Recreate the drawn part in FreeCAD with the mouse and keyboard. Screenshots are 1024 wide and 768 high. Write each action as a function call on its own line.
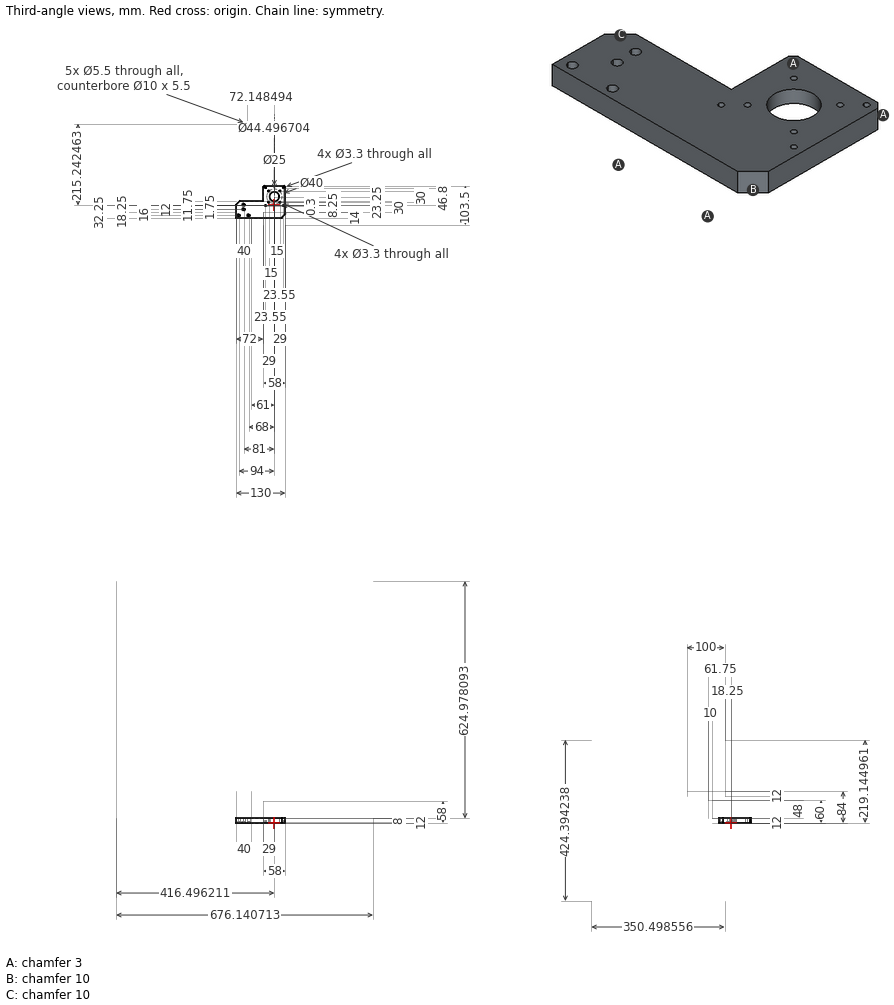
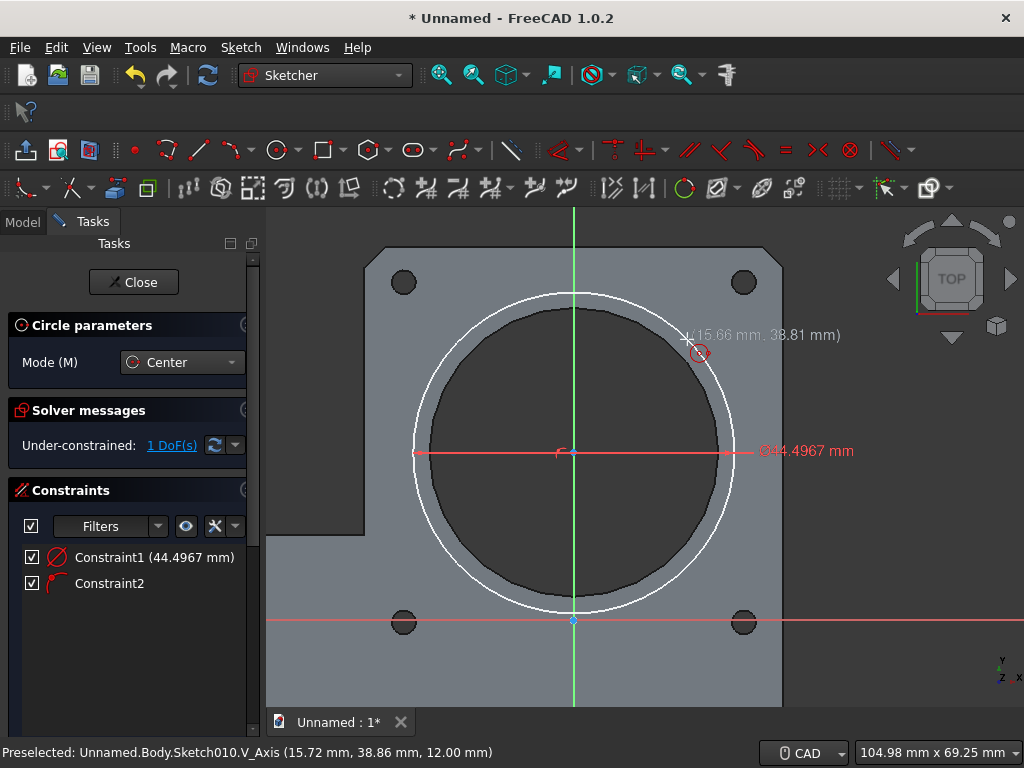
click(574, 453)
move(638, 389)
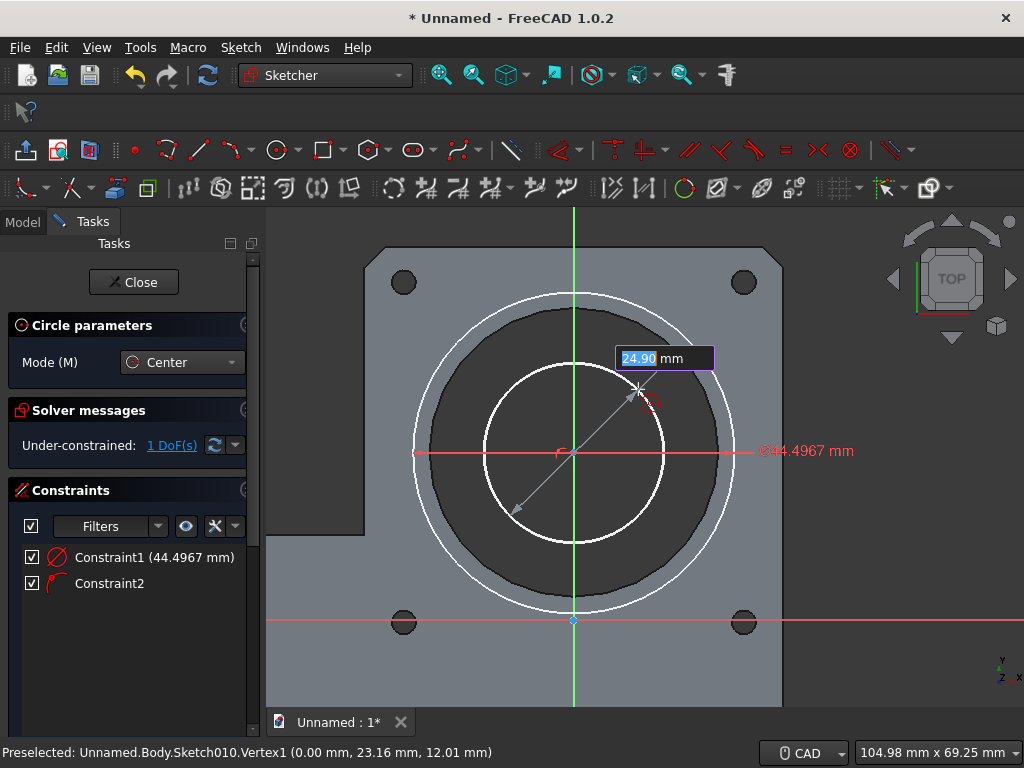
text(25)
key(Return)
key(Escape)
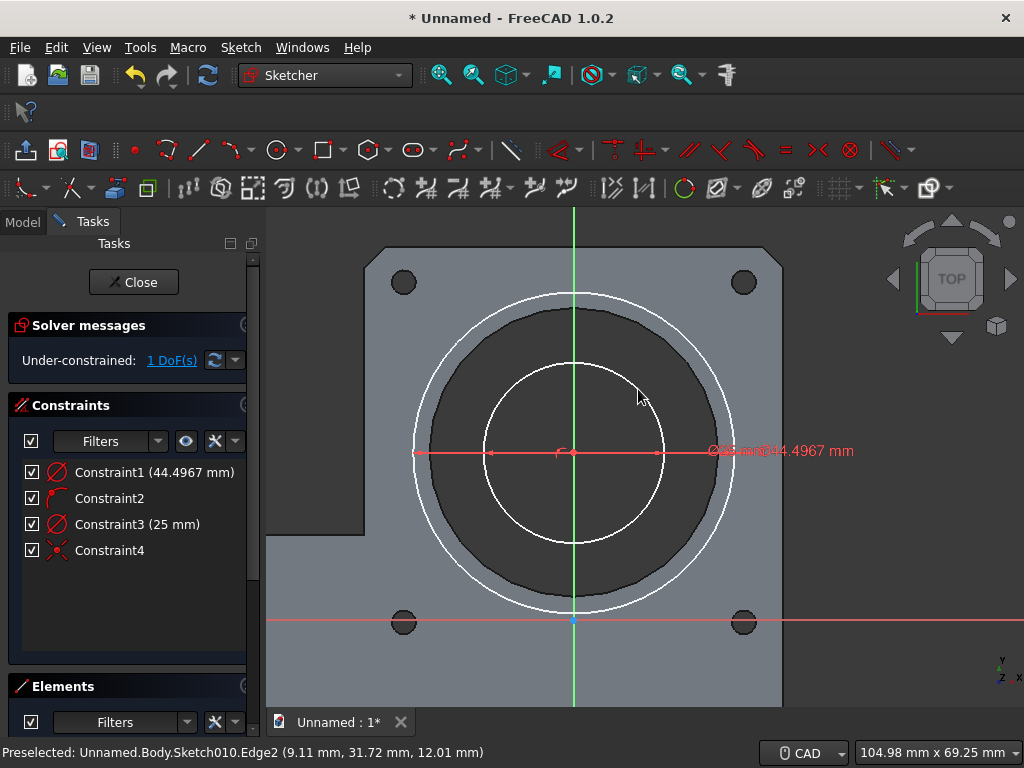
click(558, 150)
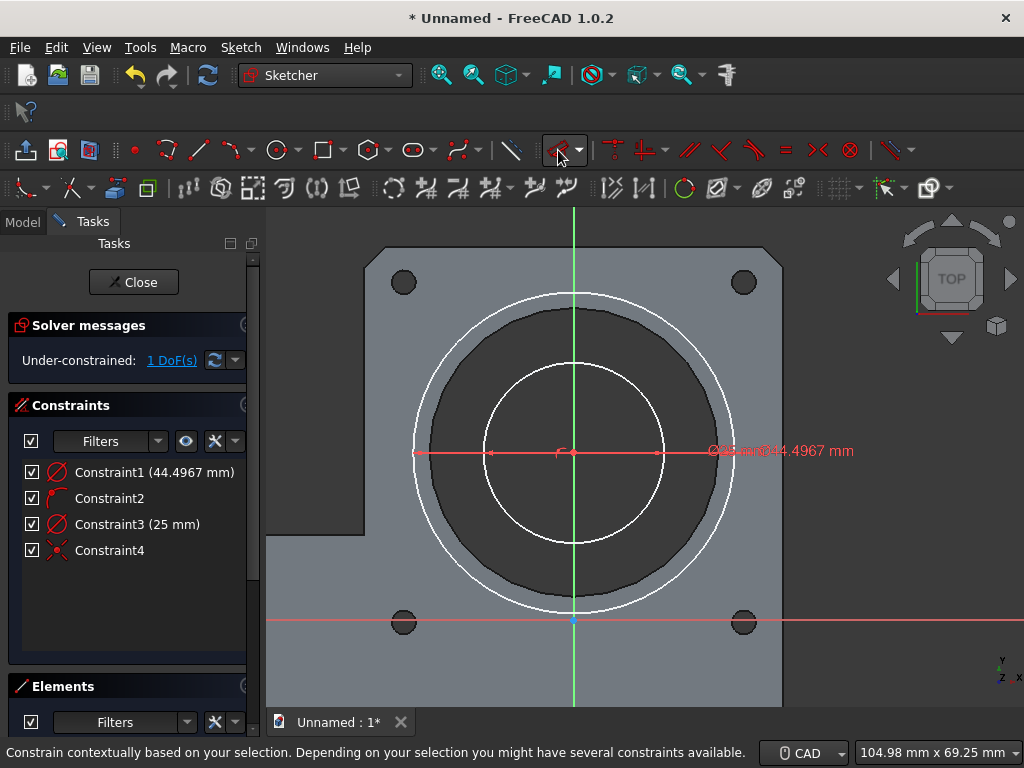
click(574, 453)
click(608, 498)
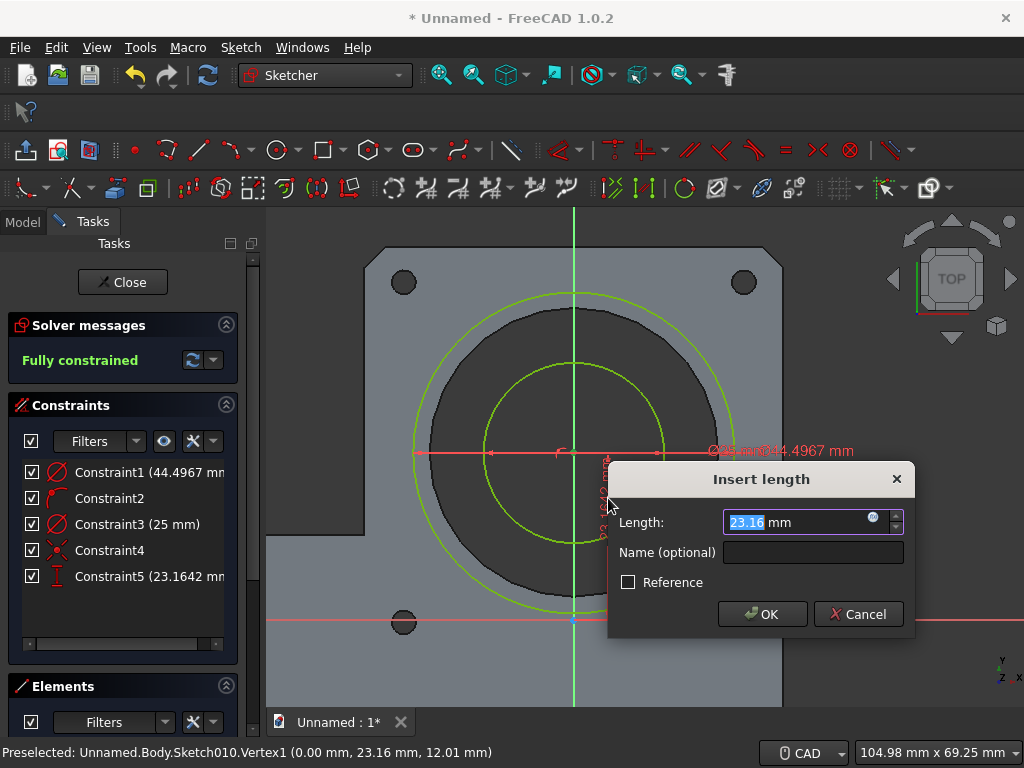
text(23.25)
key(Return)
key(Escape)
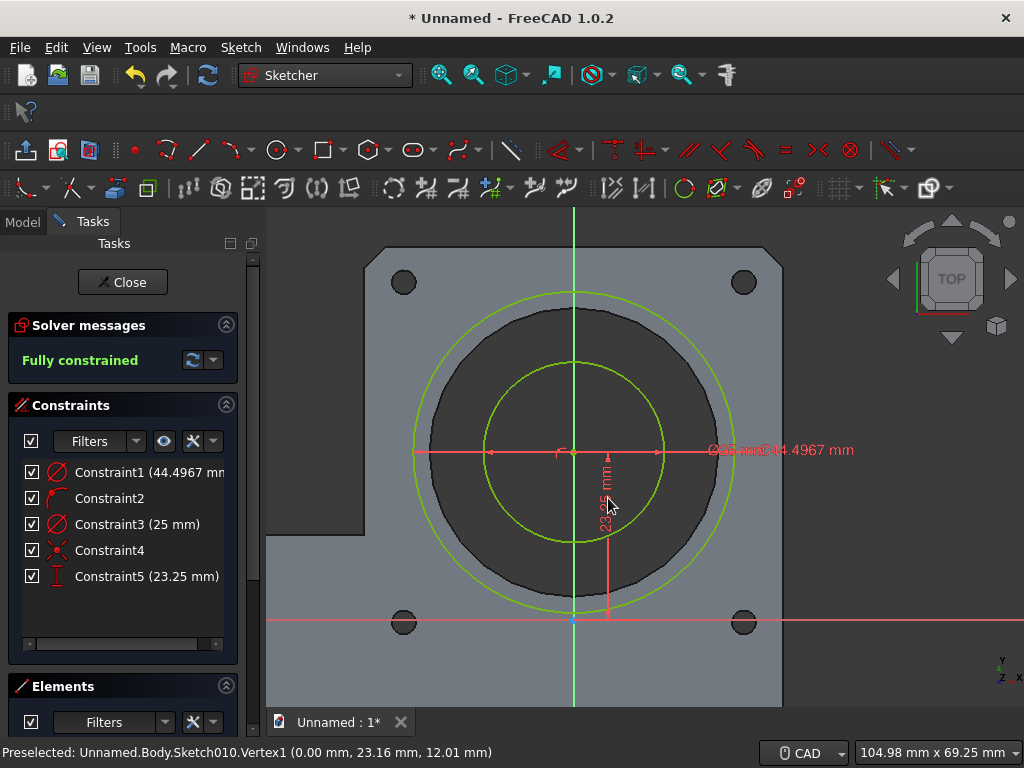
click(123, 282)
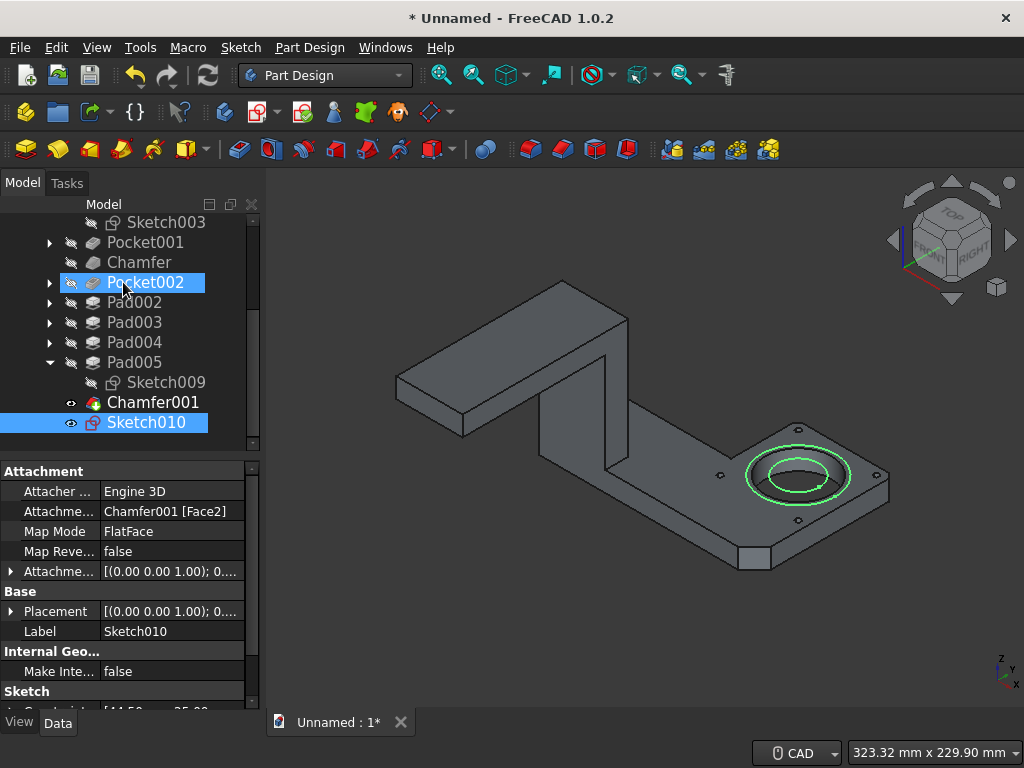
click(26, 150)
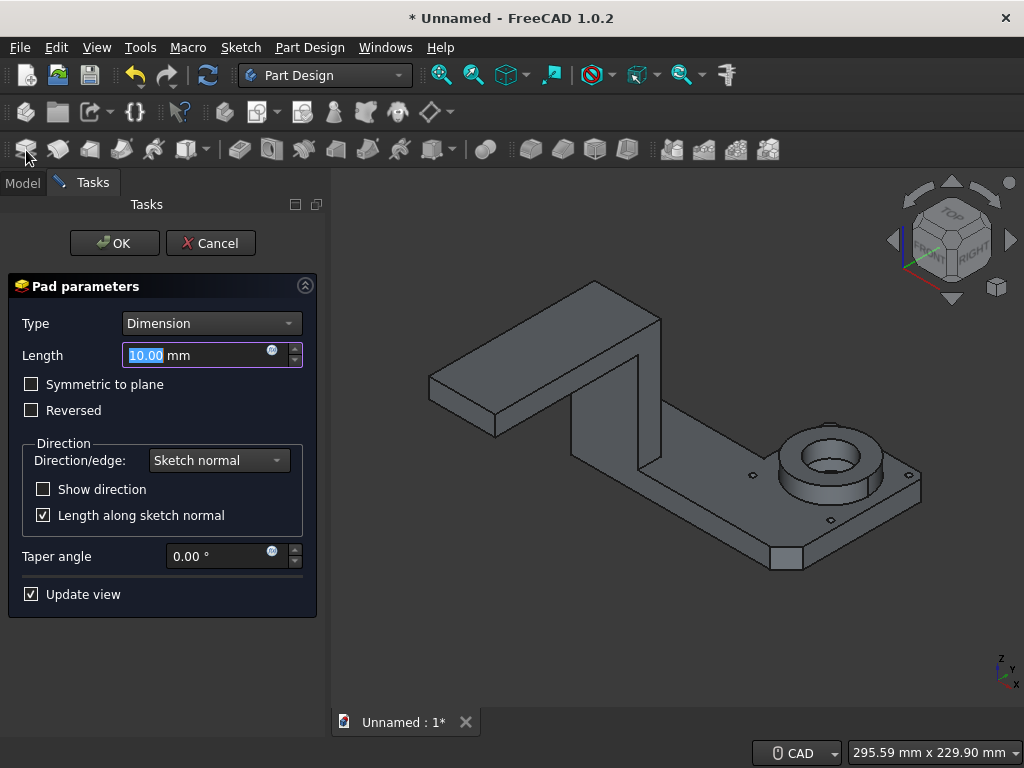
text(8)
key(Tab)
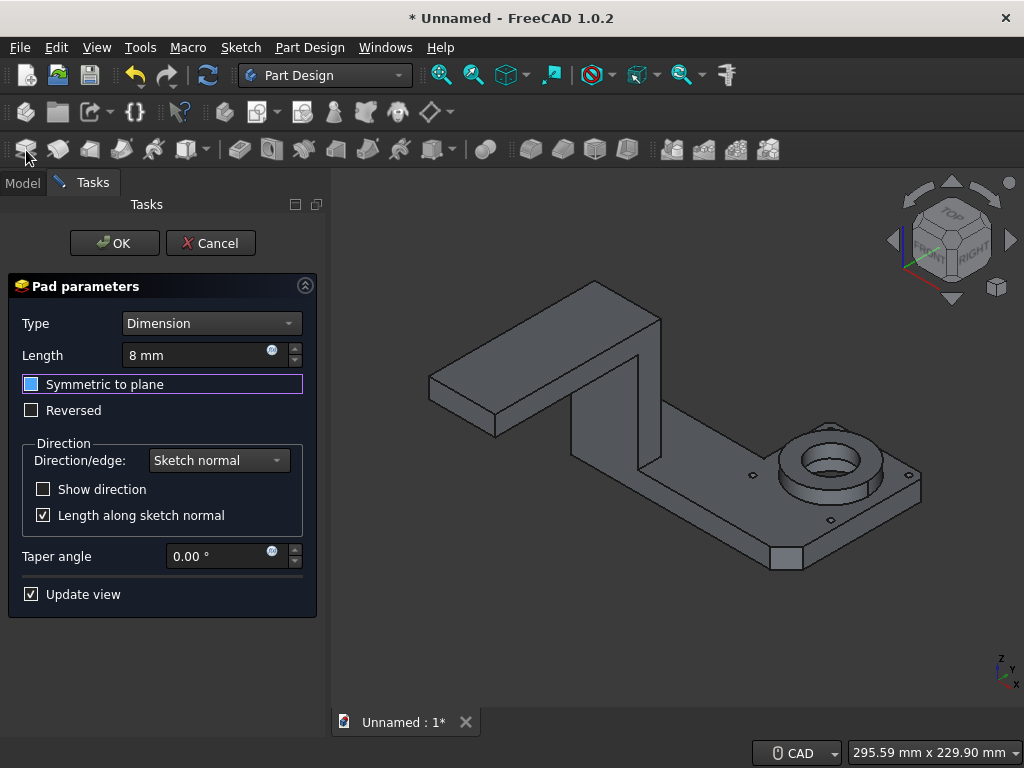
click(30, 410)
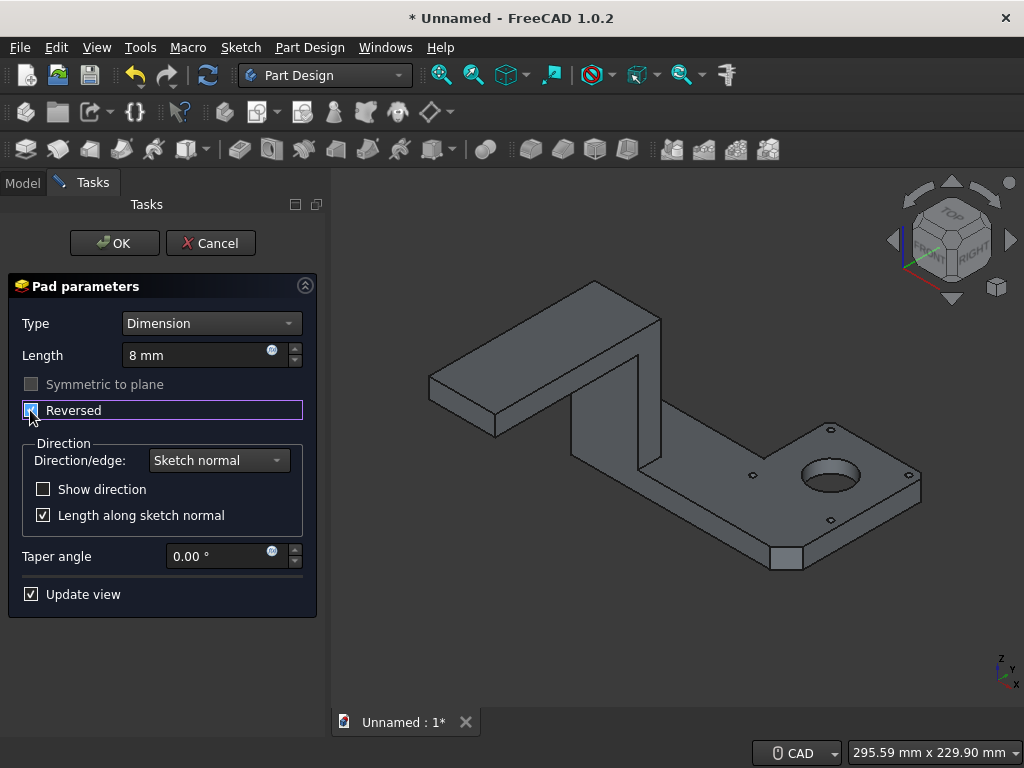
click(115, 243)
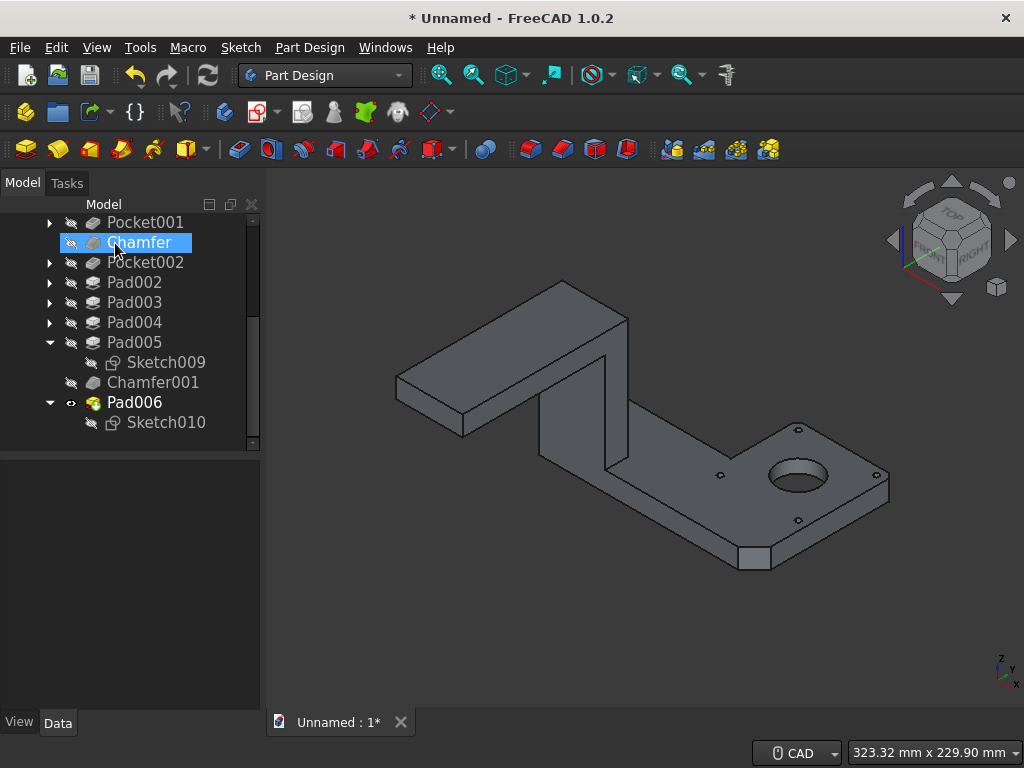
click(582, 390)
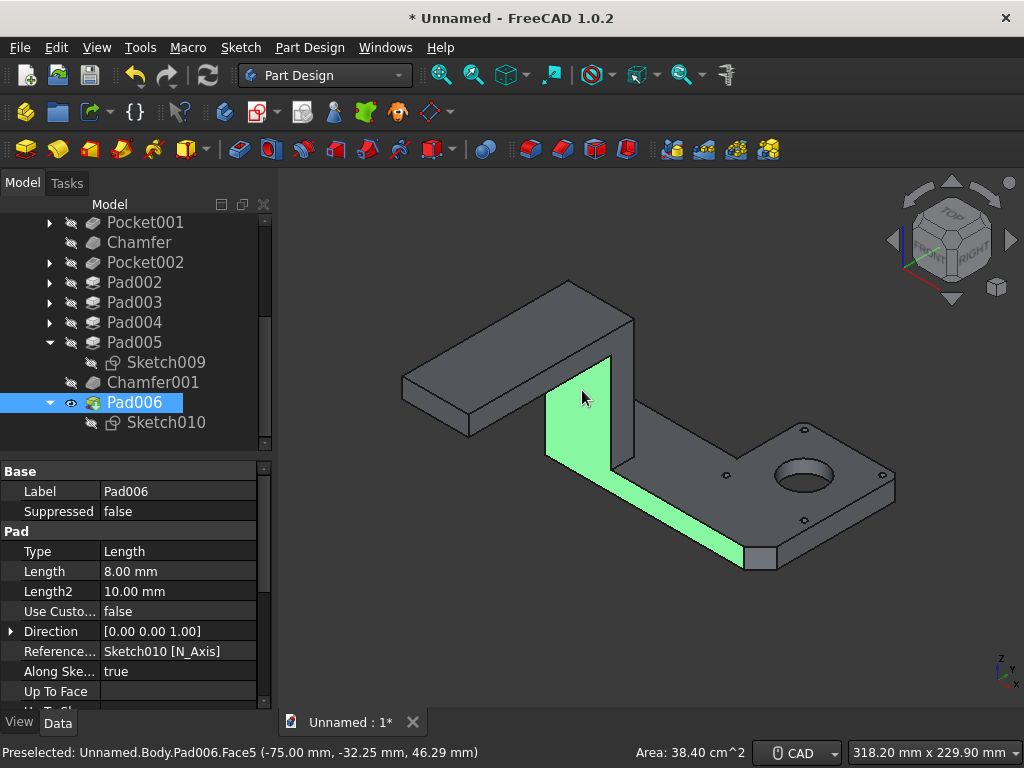
click(258, 112)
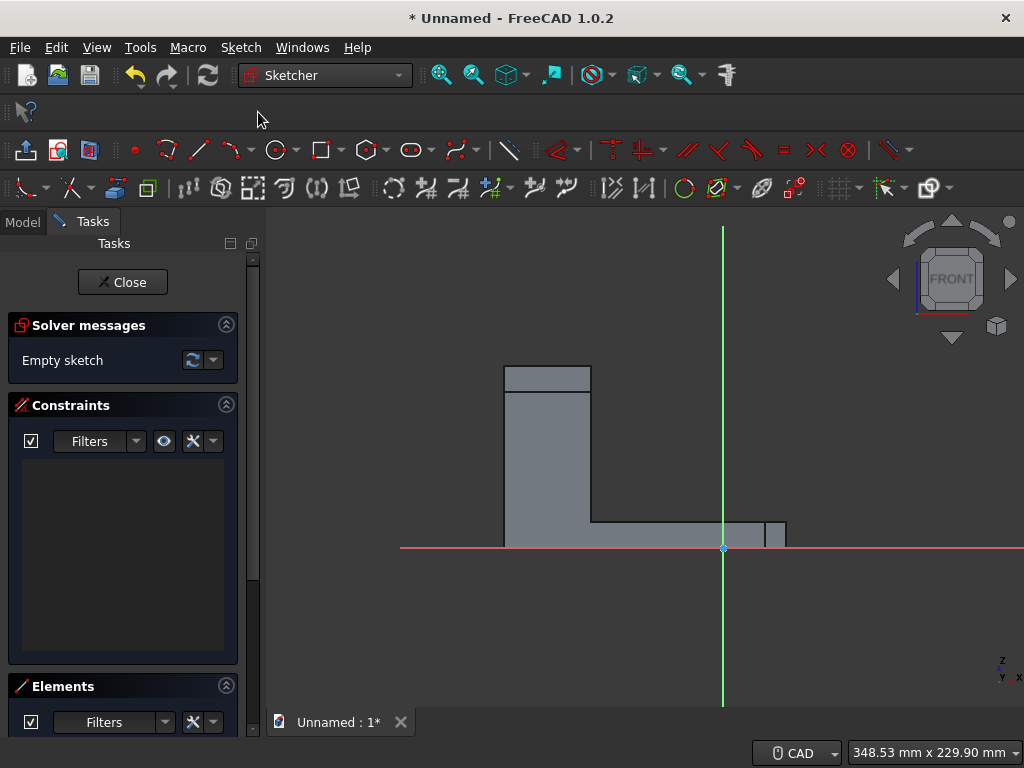
click(90, 150)